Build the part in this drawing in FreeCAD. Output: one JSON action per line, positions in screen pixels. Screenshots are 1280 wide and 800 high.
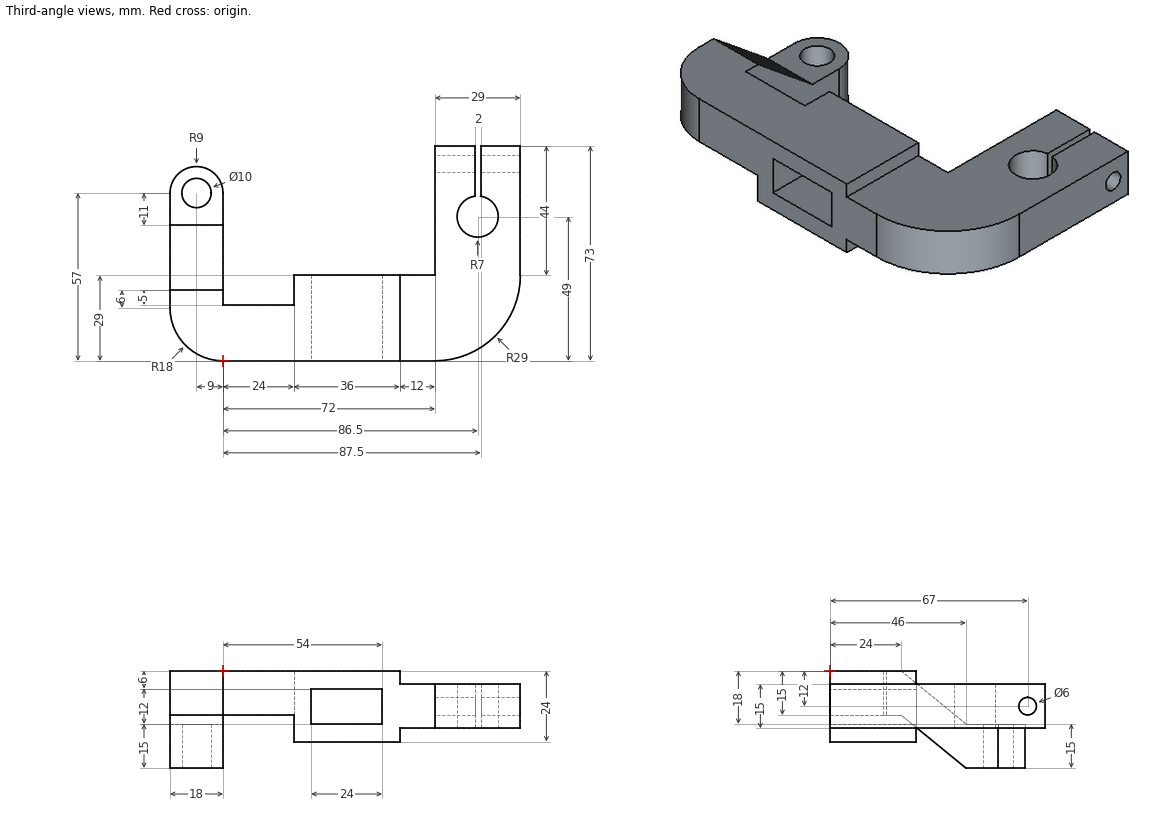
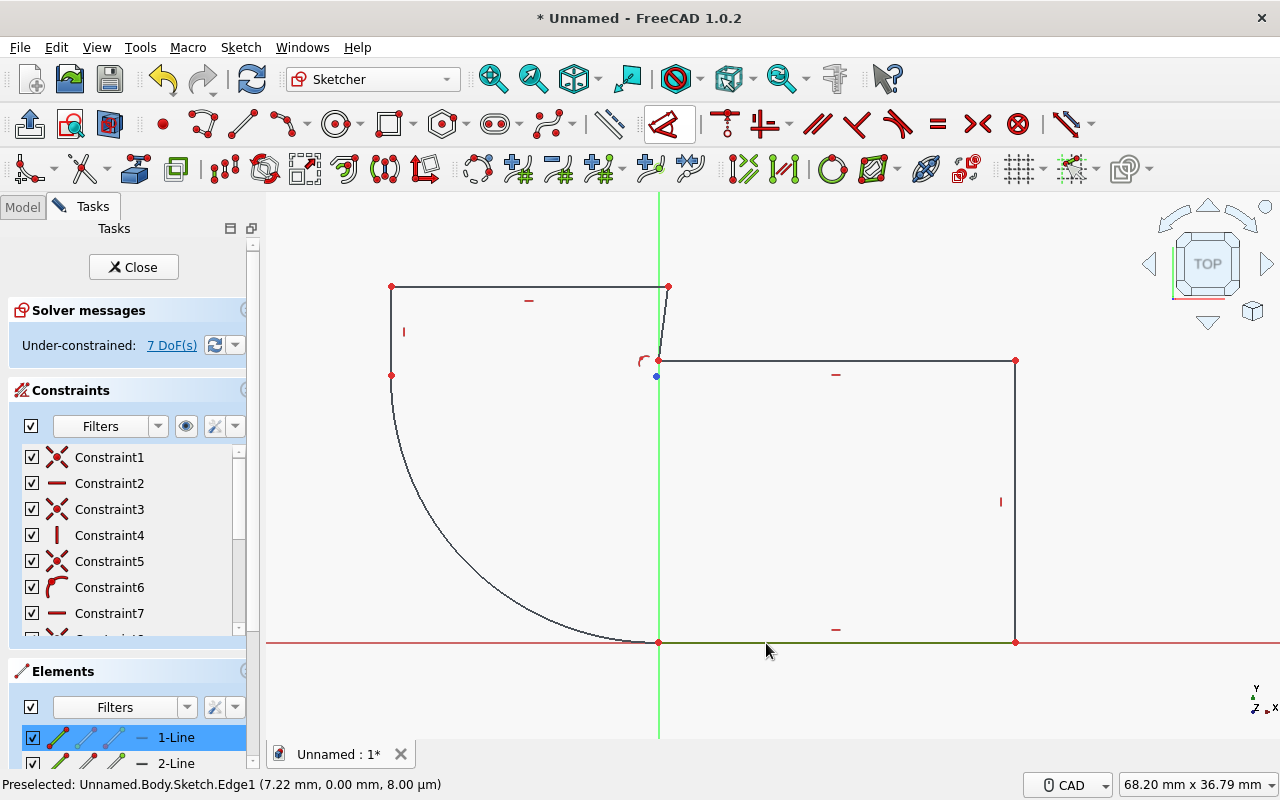
{"action": "left_click", "coordinate": [420, 498]}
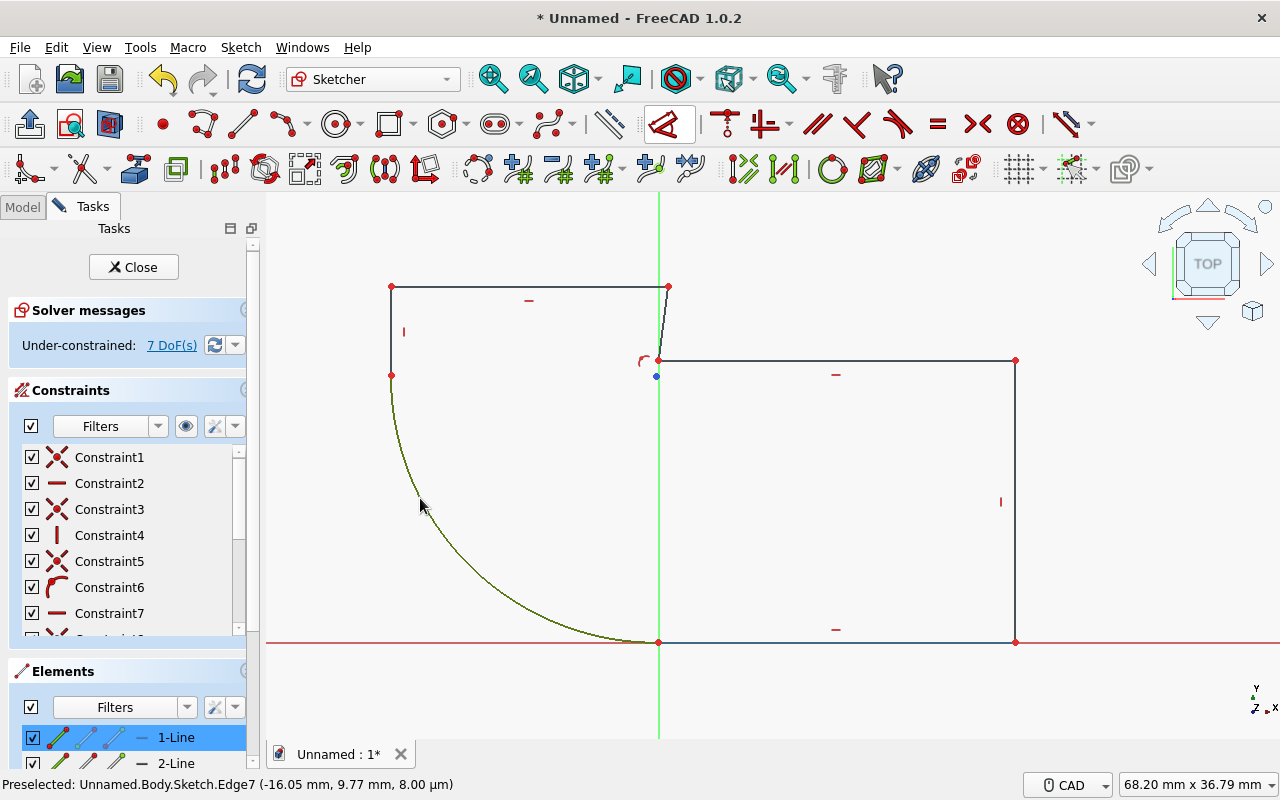
{"action": "left_click", "coordinate": [898, 124]}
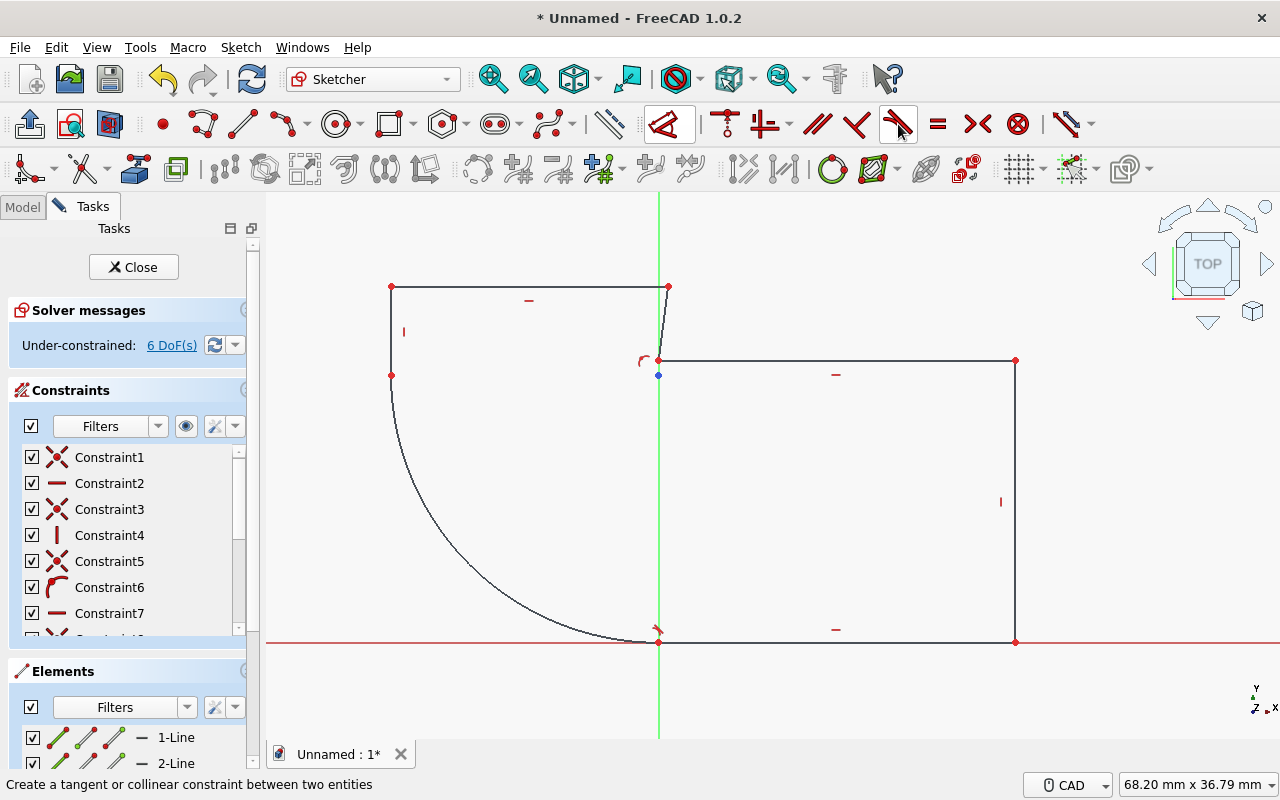
{"action": "left_click", "coordinate": [391, 314]}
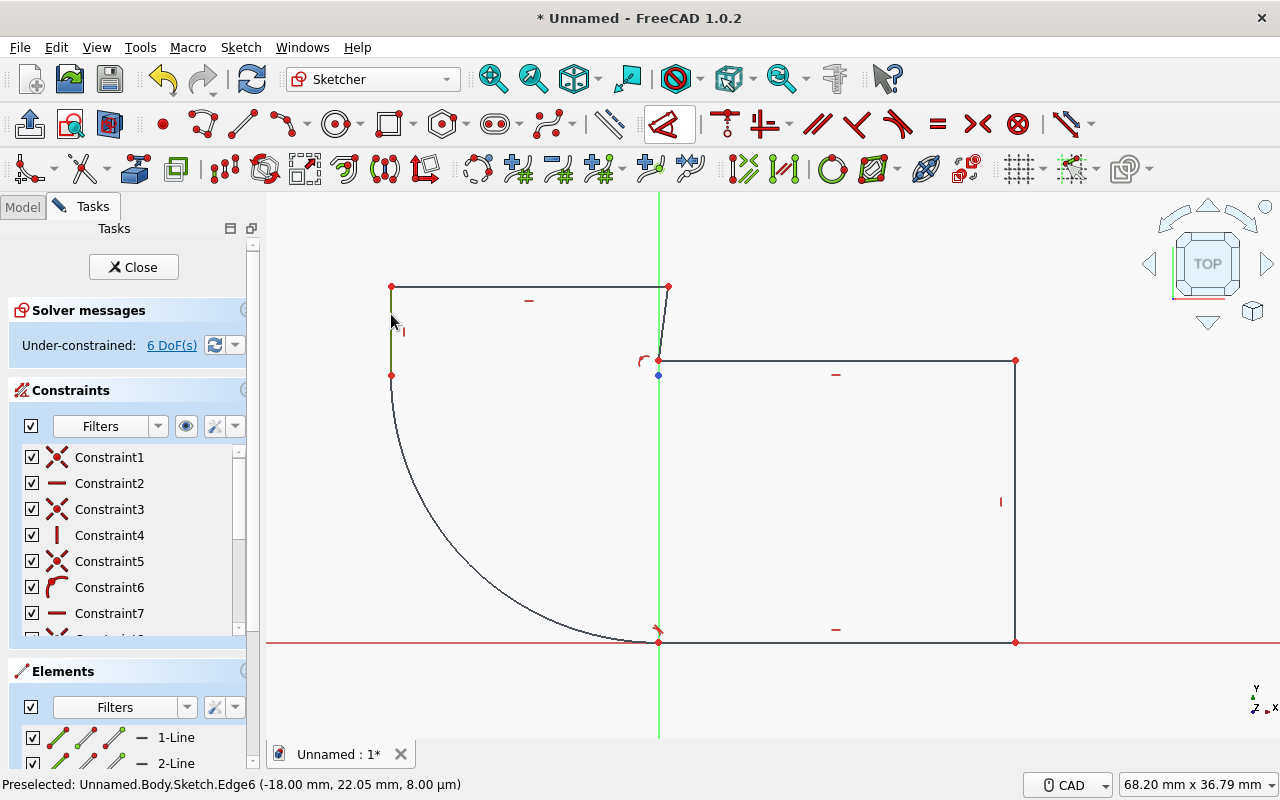
{"action": "left_click", "coordinate": [420, 497]}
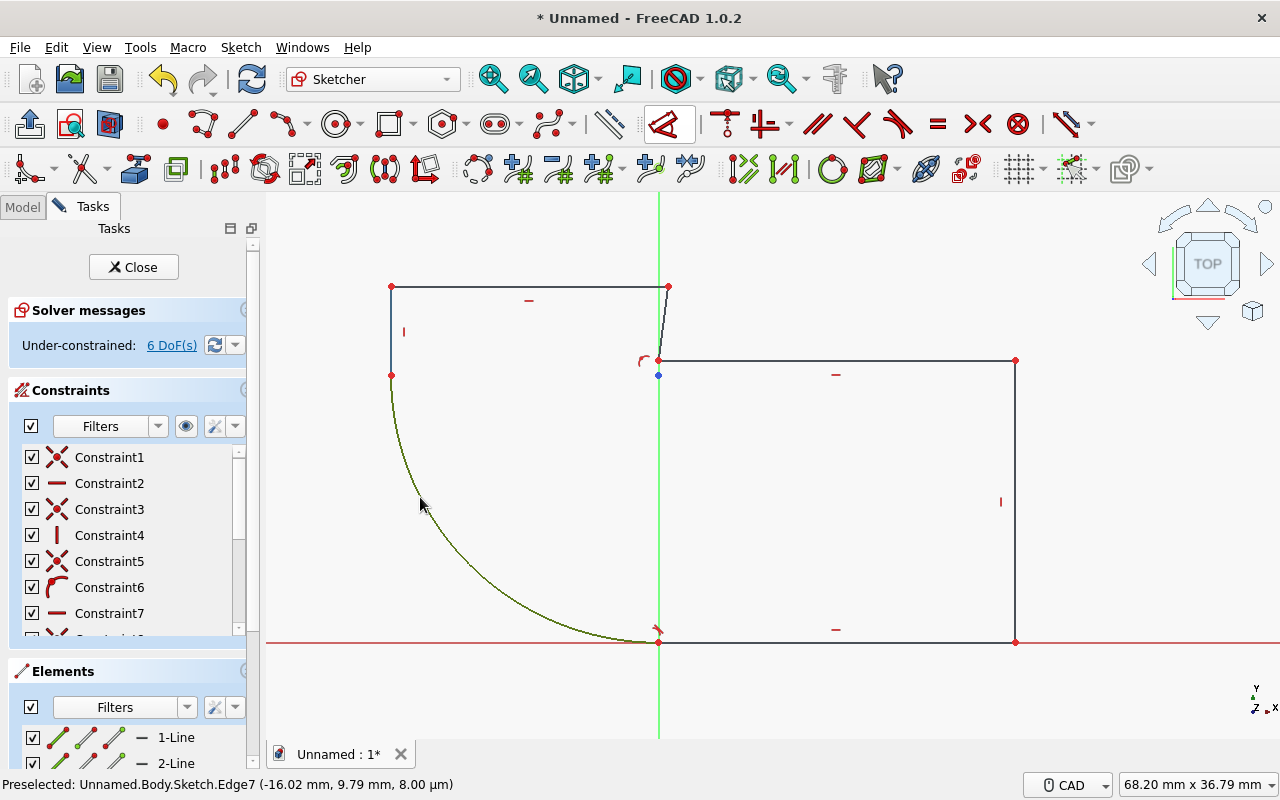
{"action": "key", "text": "t"}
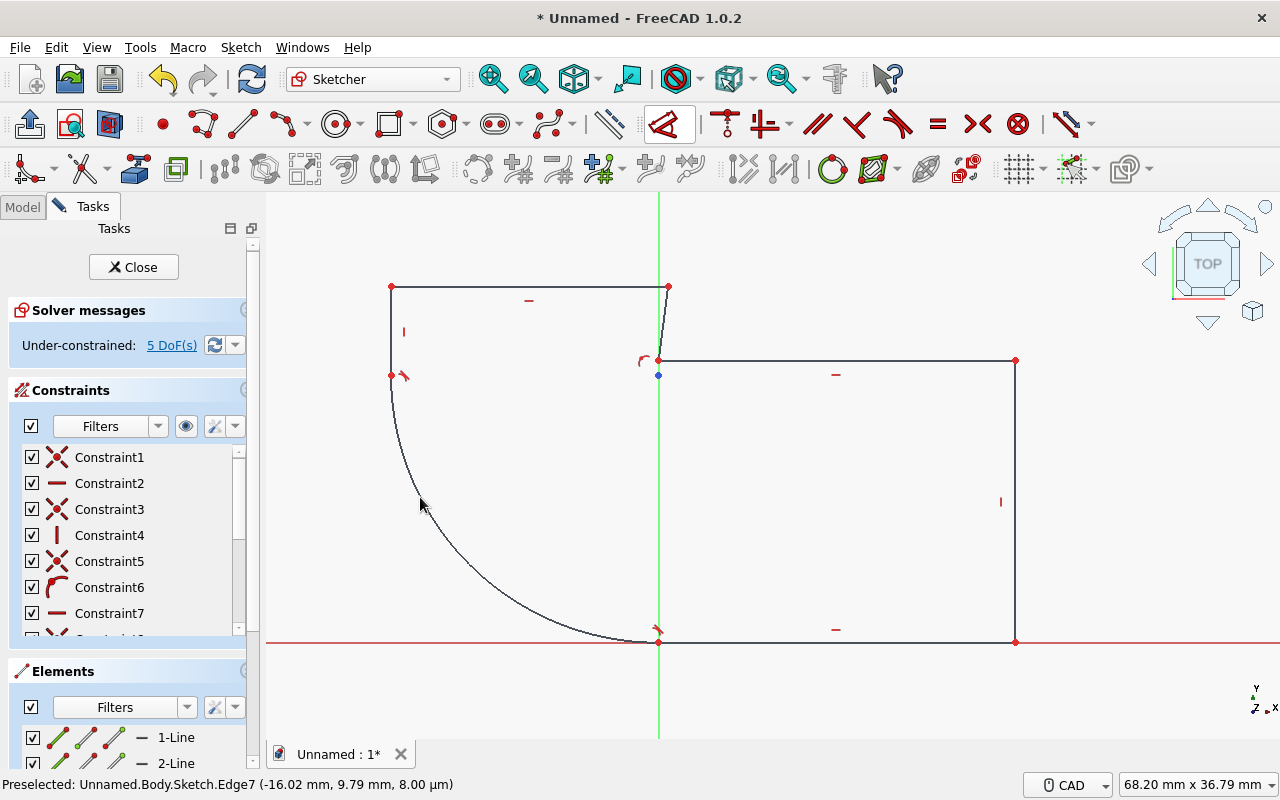
{"action": "left_click", "coordinate": [661, 339]}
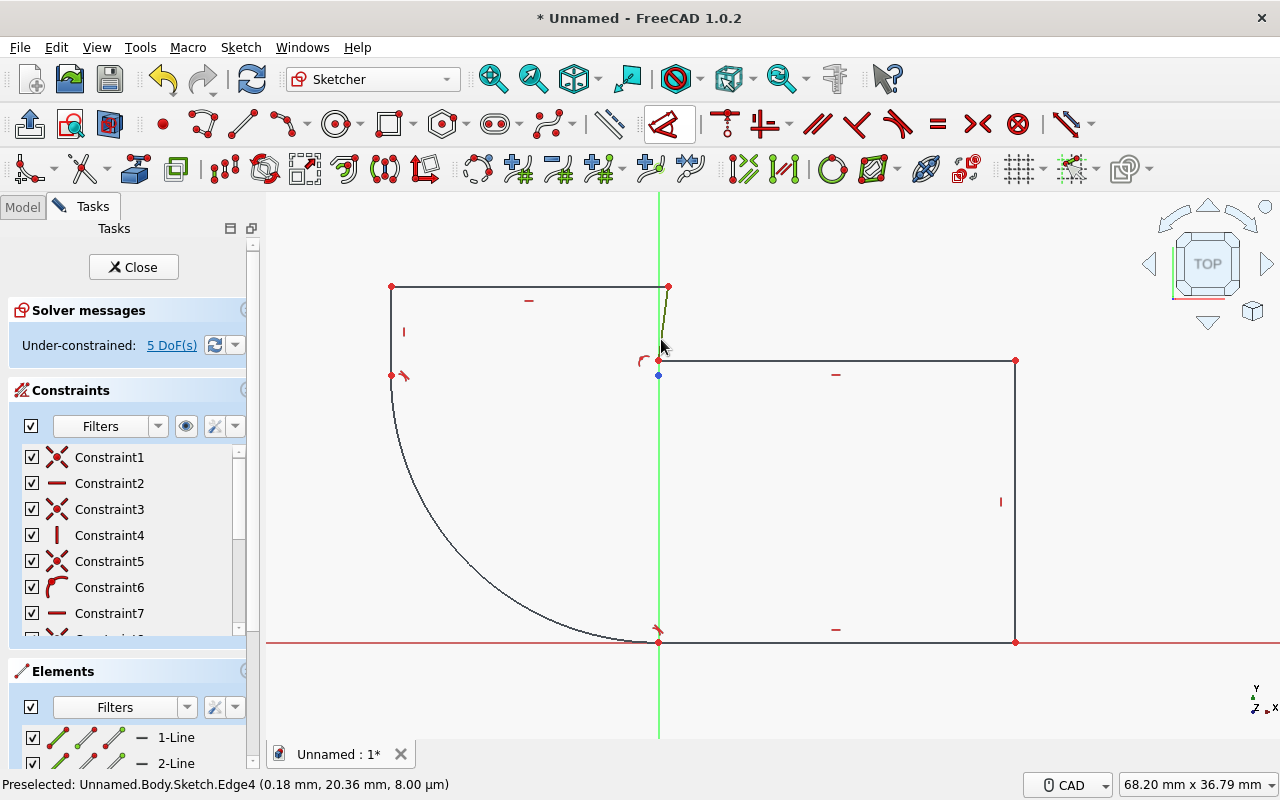
{"action": "left_click", "coordinate": [792, 124]}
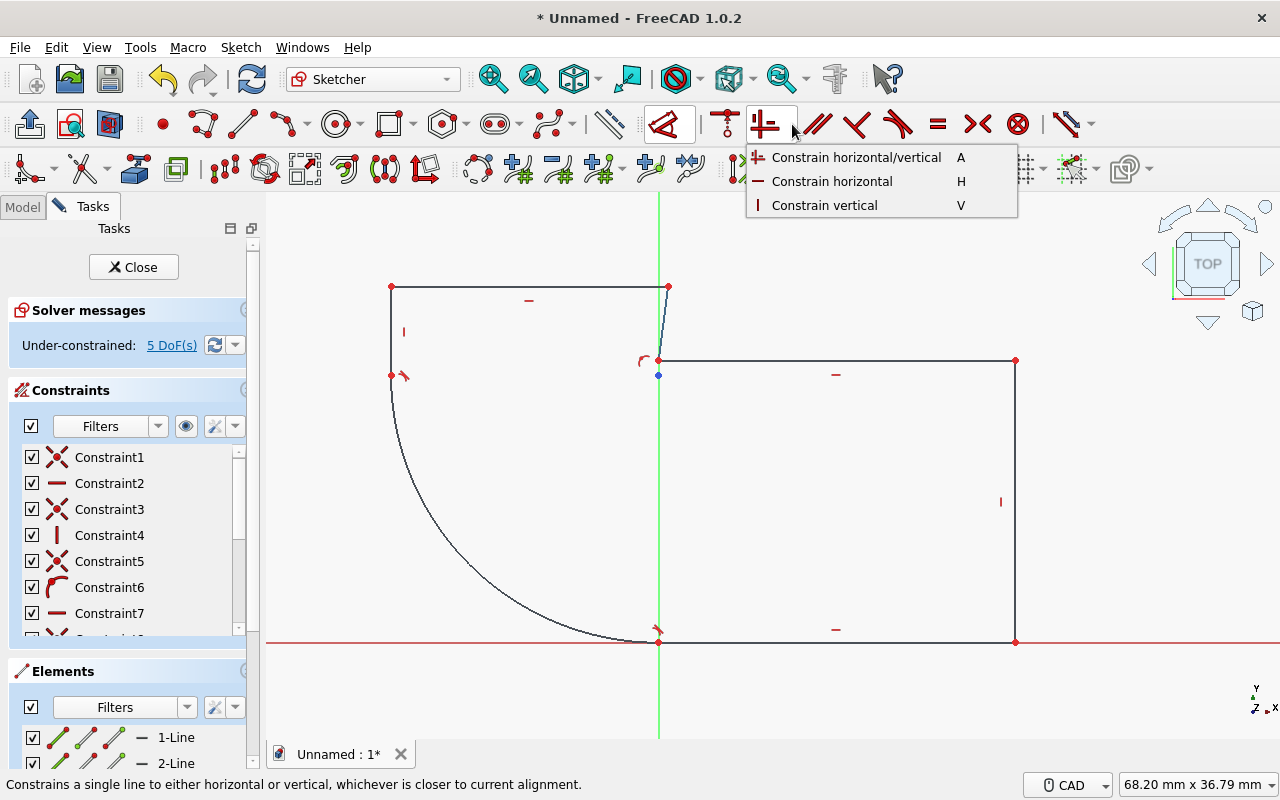
{"action": "left_click", "coordinate": [882, 205]}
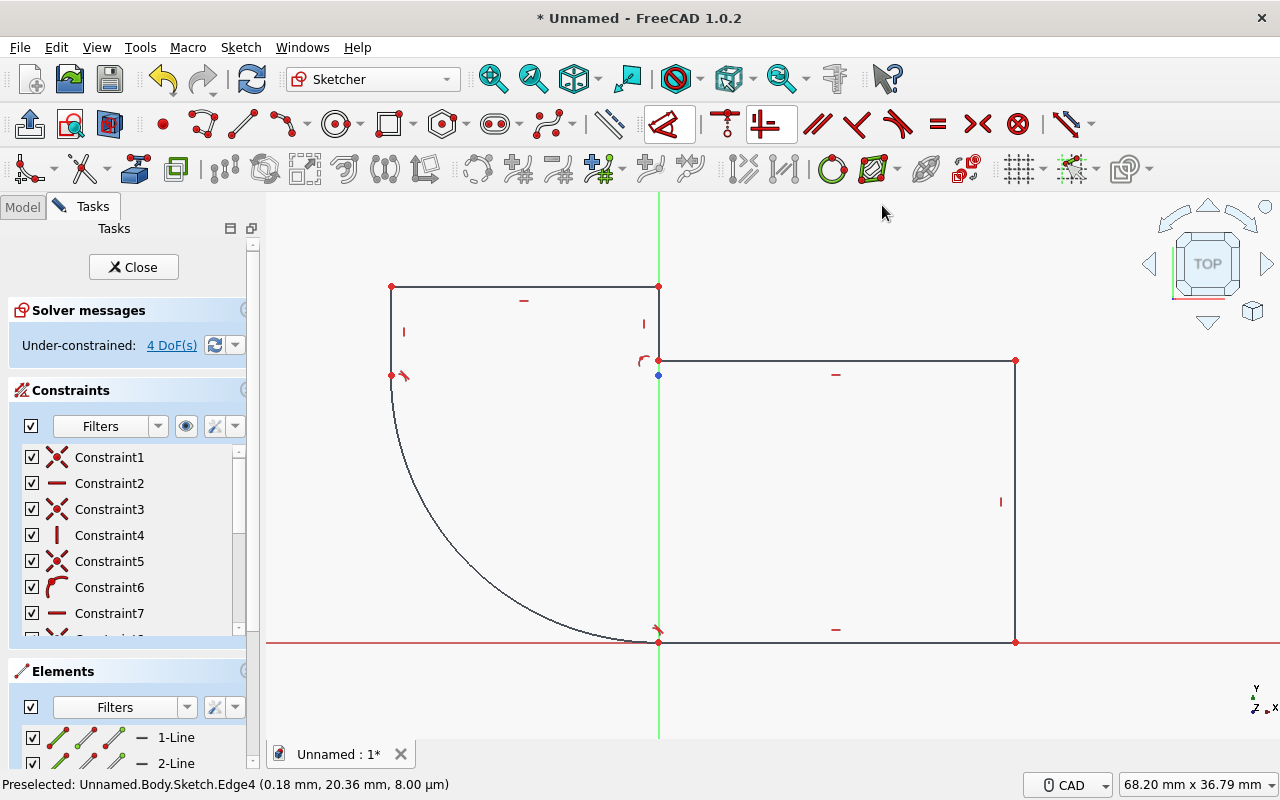
{"action": "left_click", "coordinate": [664, 124]}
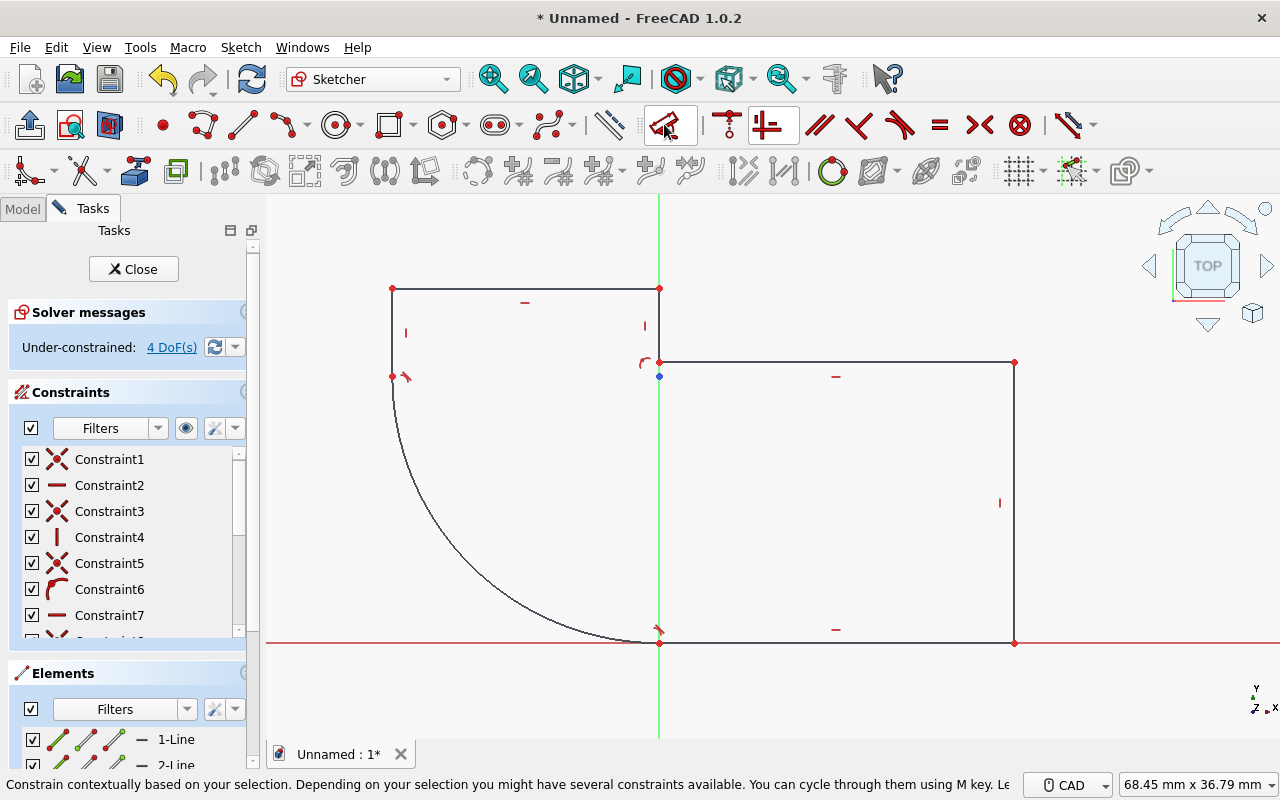
{"action": "left_click", "coordinate": [421, 498]}
{"action": "left_click", "coordinate": [392, 513]}